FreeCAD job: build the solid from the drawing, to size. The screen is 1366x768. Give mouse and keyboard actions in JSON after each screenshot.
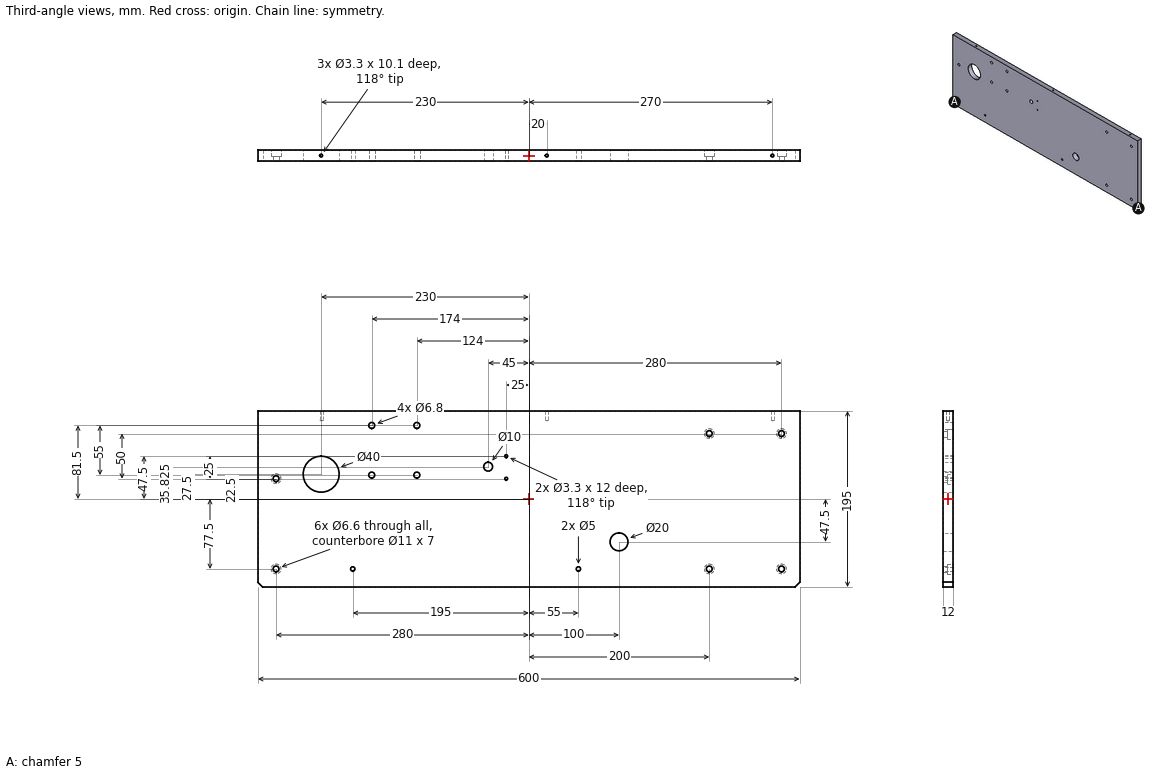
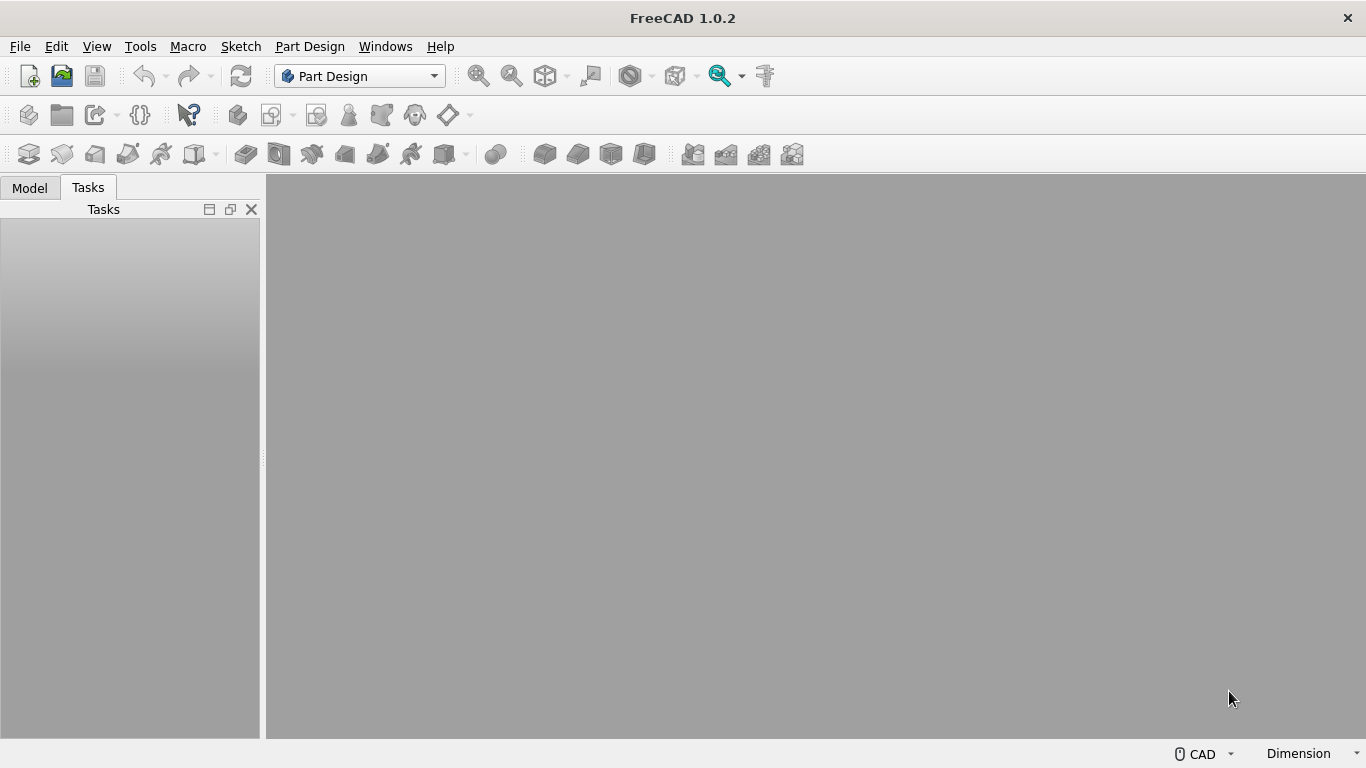
{"action": "left_click", "coordinate": [29, 76]}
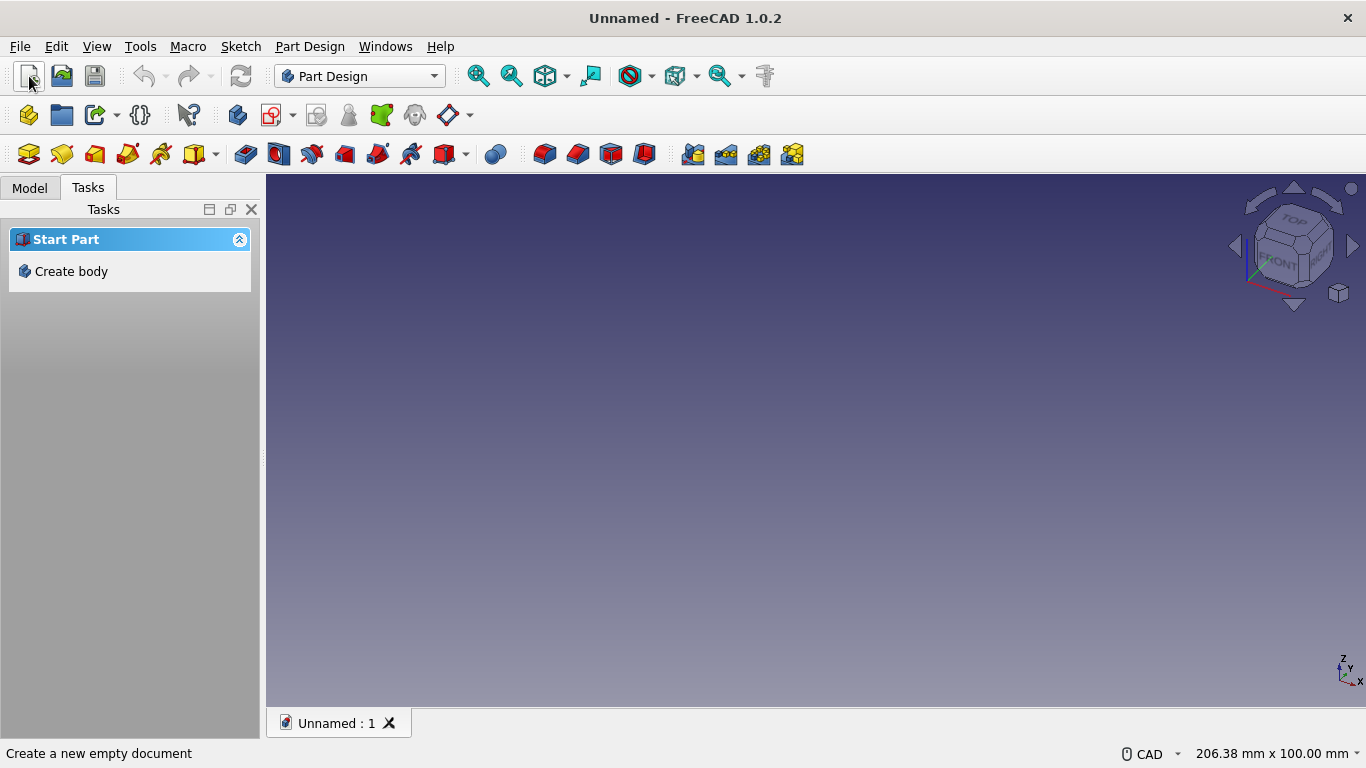
{"action": "left_click", "coordinate": [270, 116]}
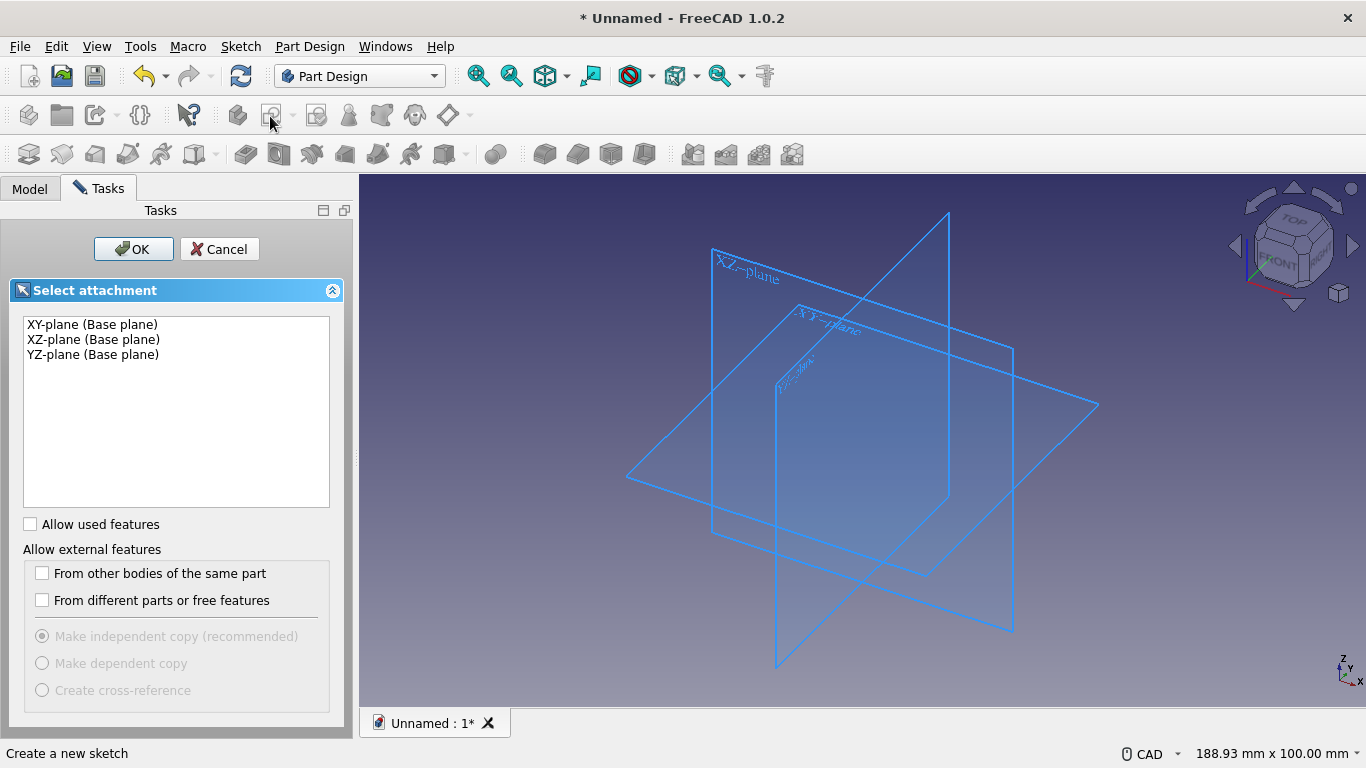
{"action": "left_click", "coordinate": [84, 340]}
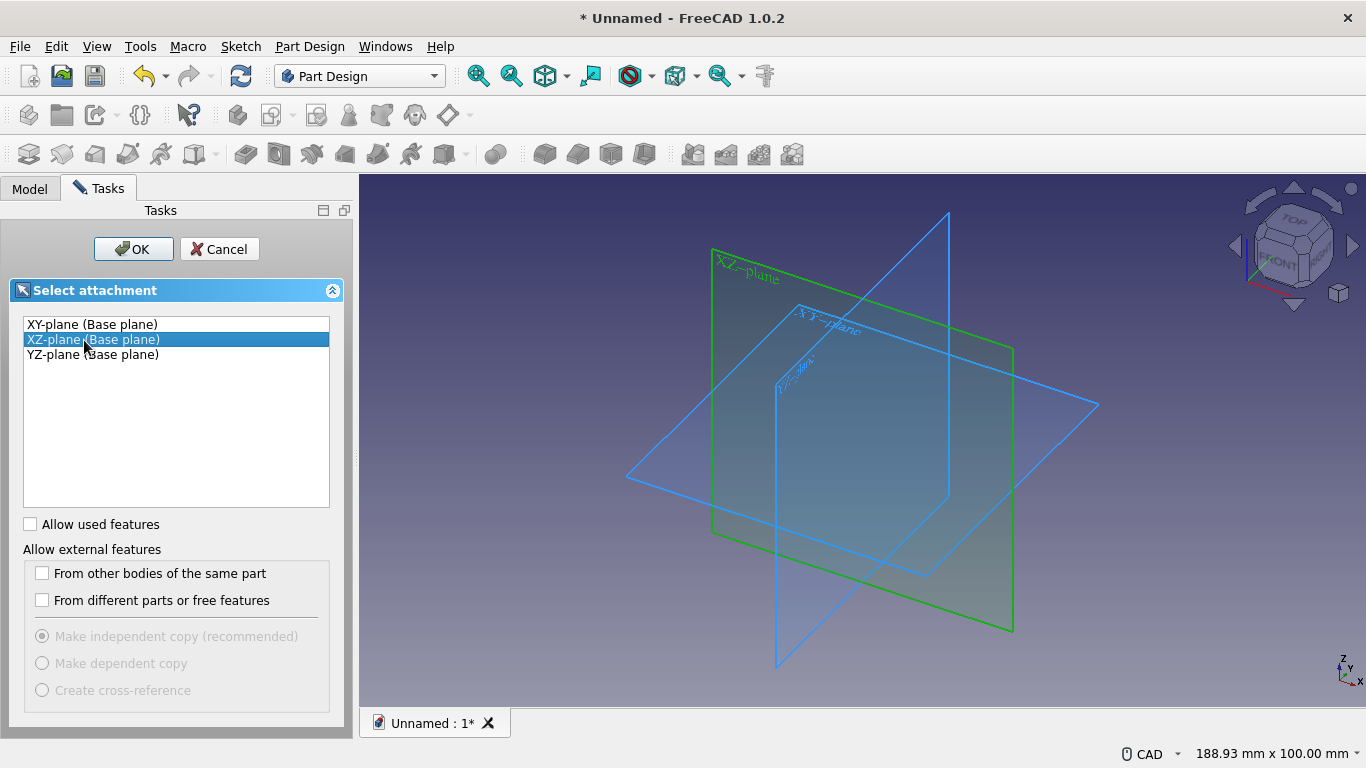
{"action": "left_click", "coordinate": [134, 249]}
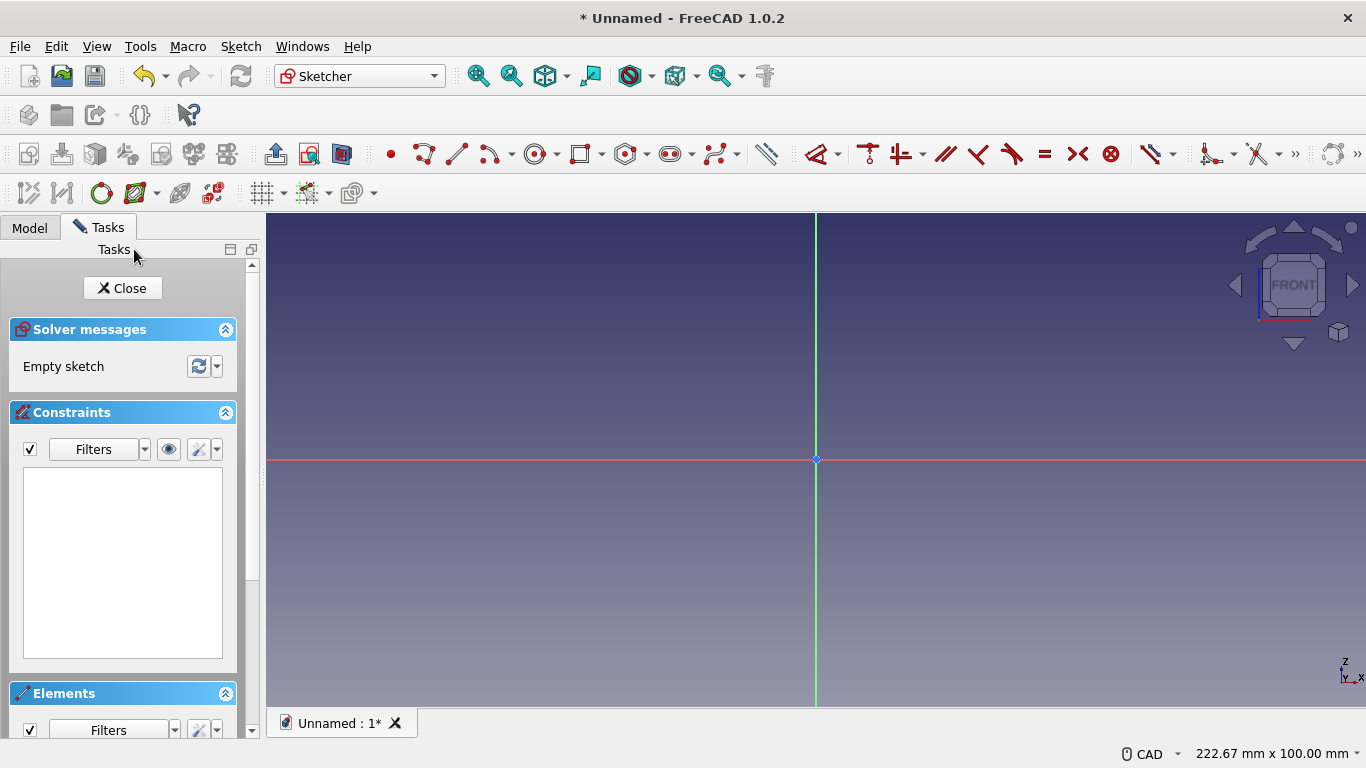
{"action": "scroll", "coordinate": [730, 460], "scroll_direction": "down", "scroll_amount": 8}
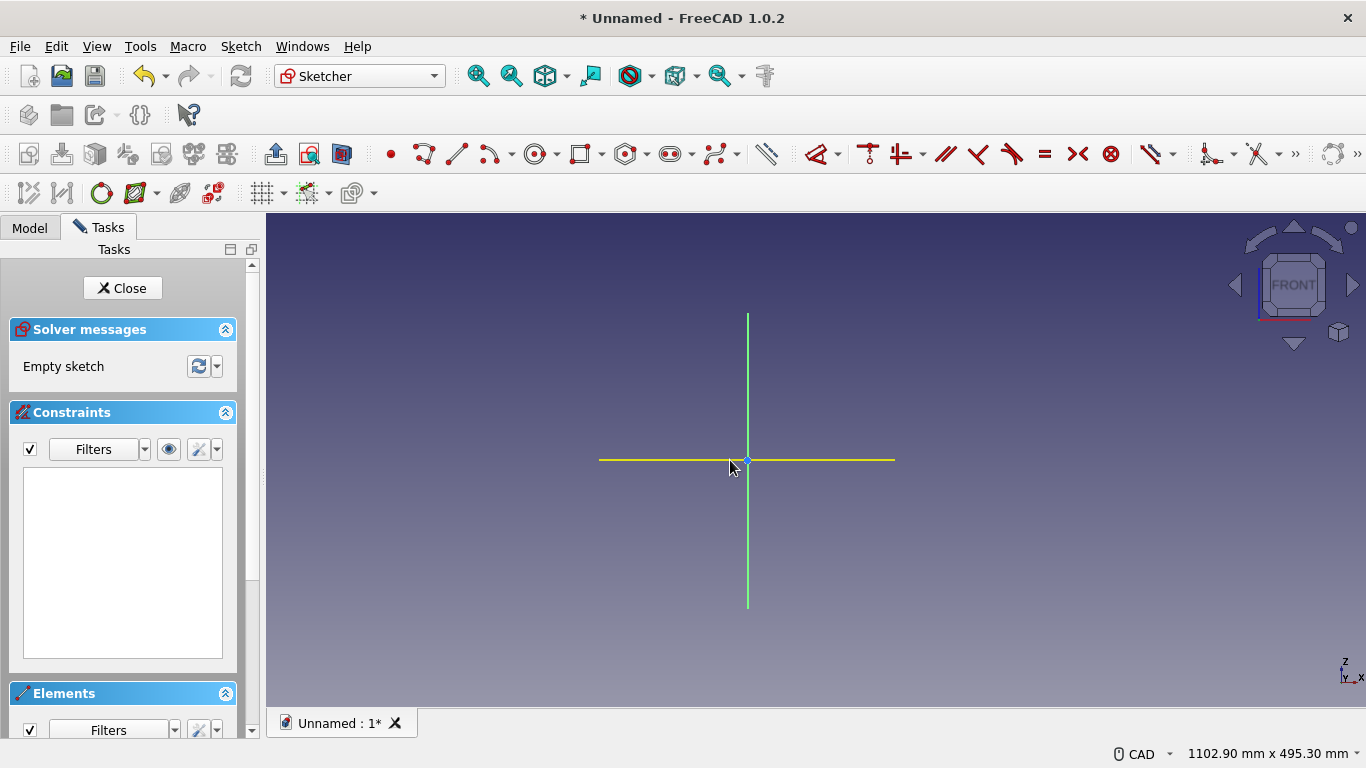
{"action": "left_click", "coordinate": [602, 154]}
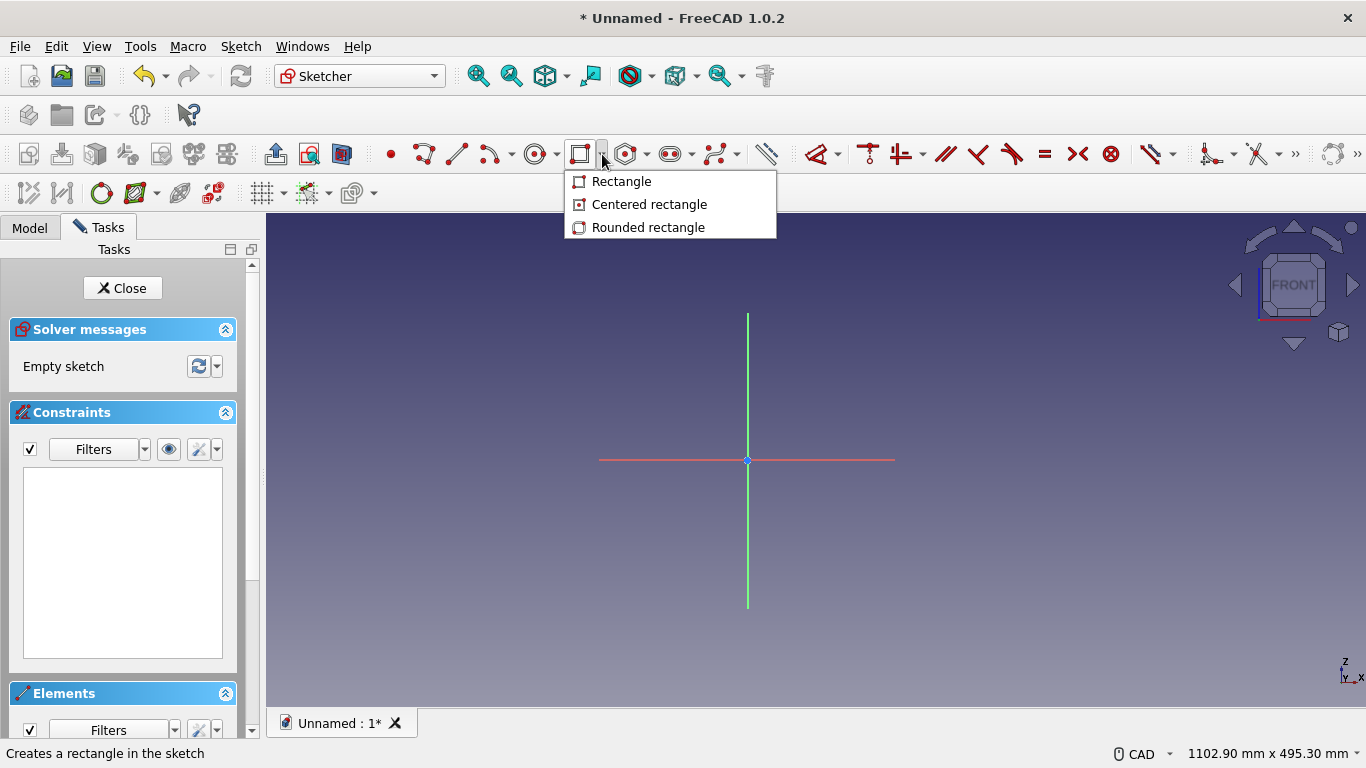
{"action": "left_click", "coordinate": [670, 204]}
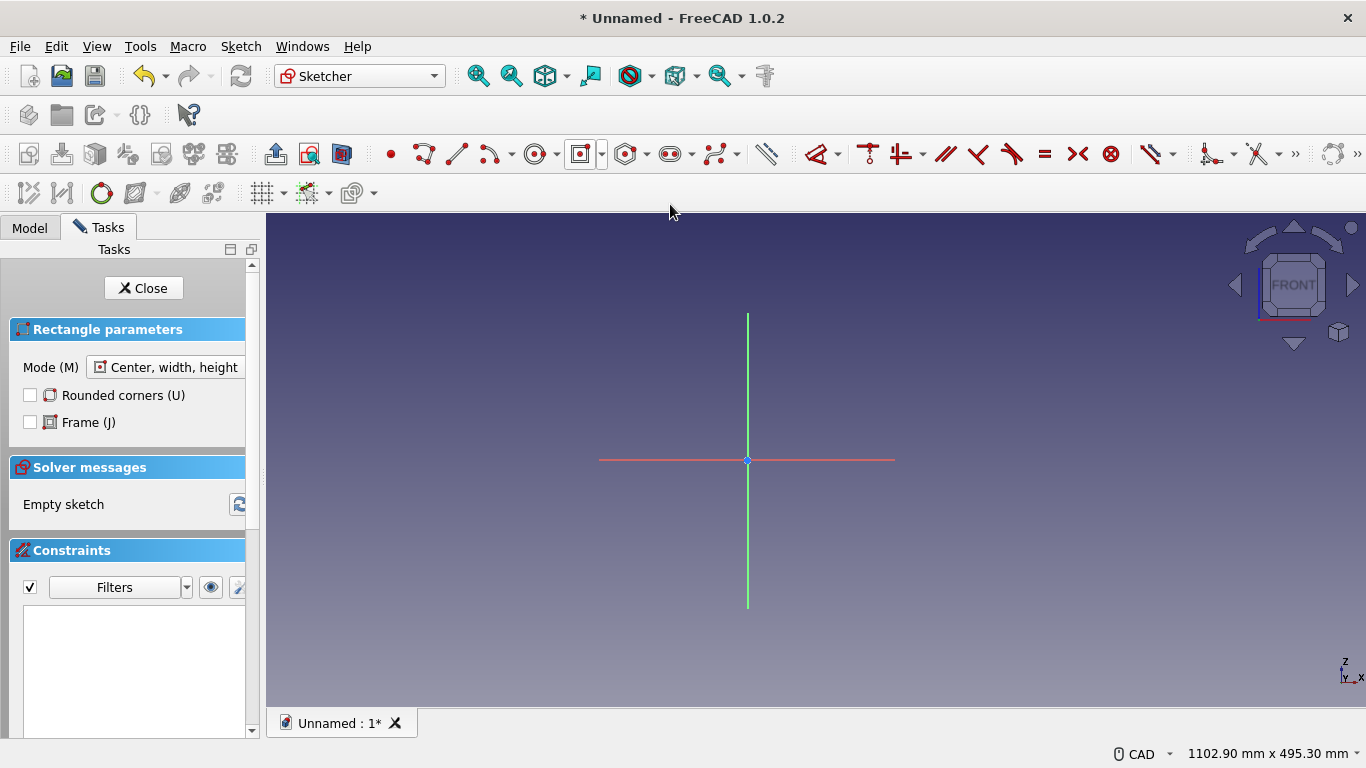
{"action": "left_click", "coordinate": [748, 460]}
{"action": "left_click", "coordinate": [1047, 363]}
{"action": "key", "text": "Escape"}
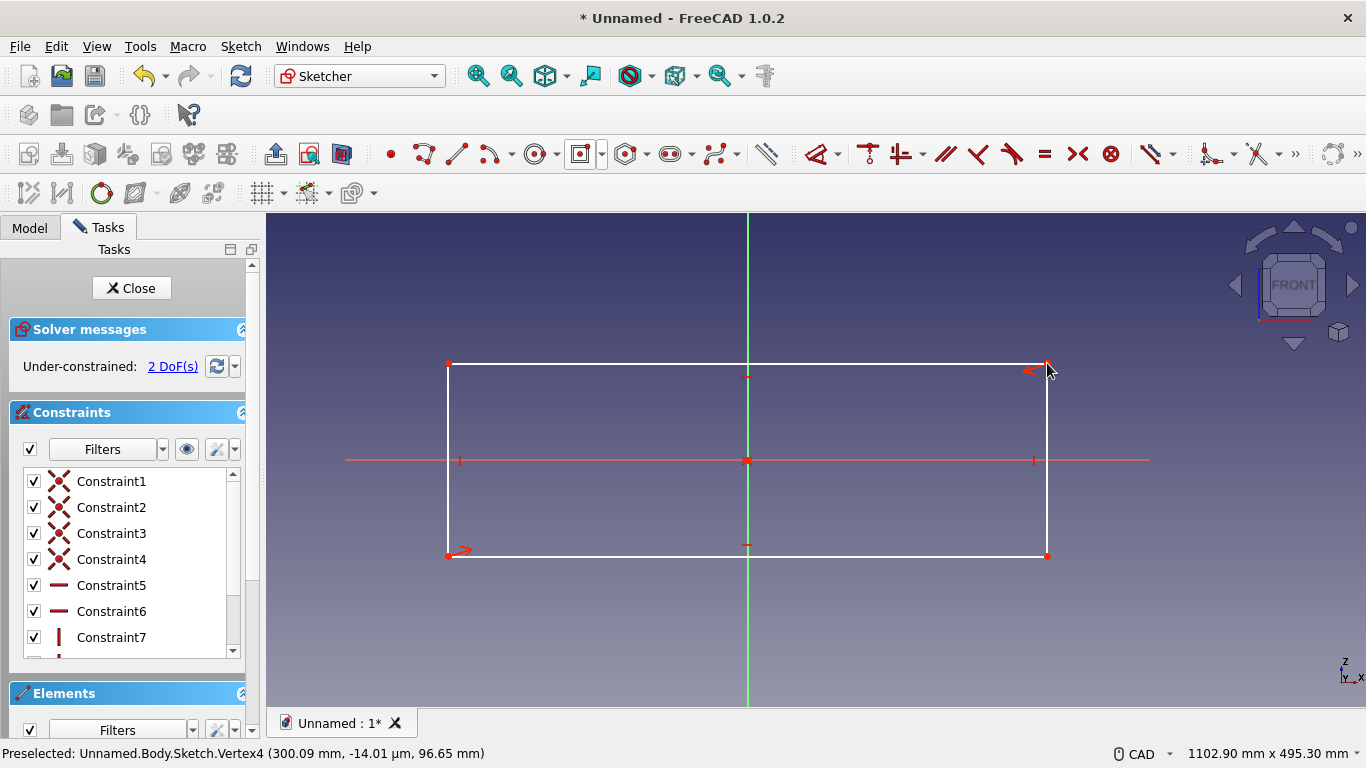
{"action": "key", "text": "d"}